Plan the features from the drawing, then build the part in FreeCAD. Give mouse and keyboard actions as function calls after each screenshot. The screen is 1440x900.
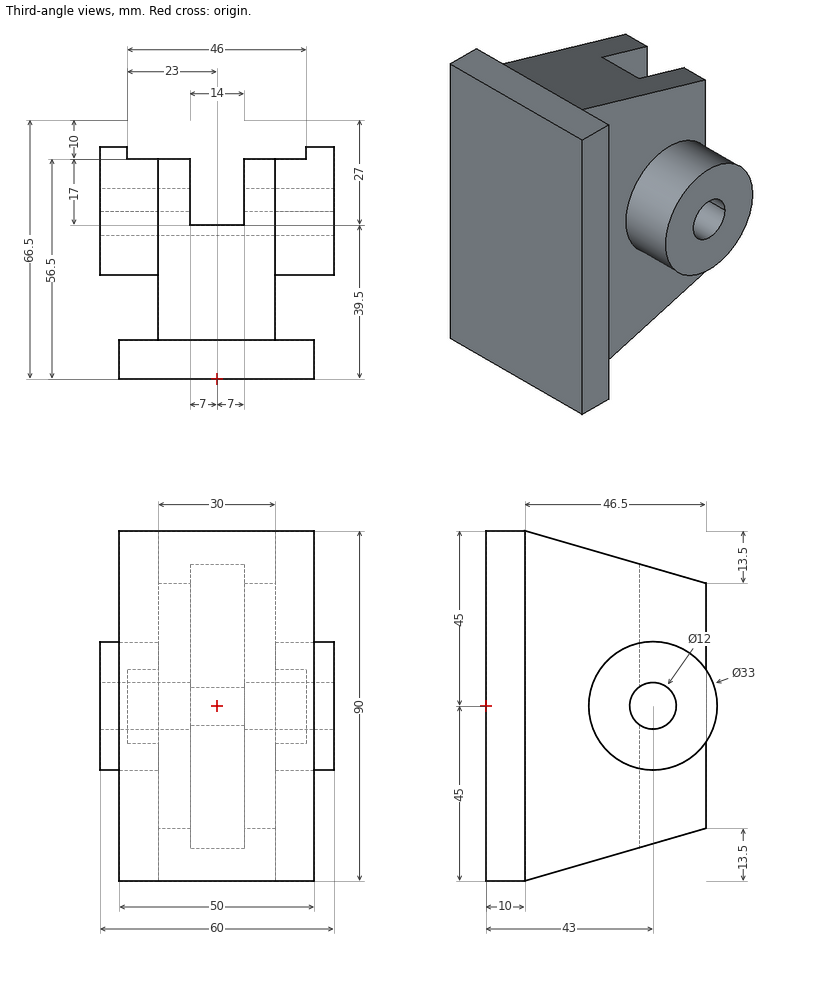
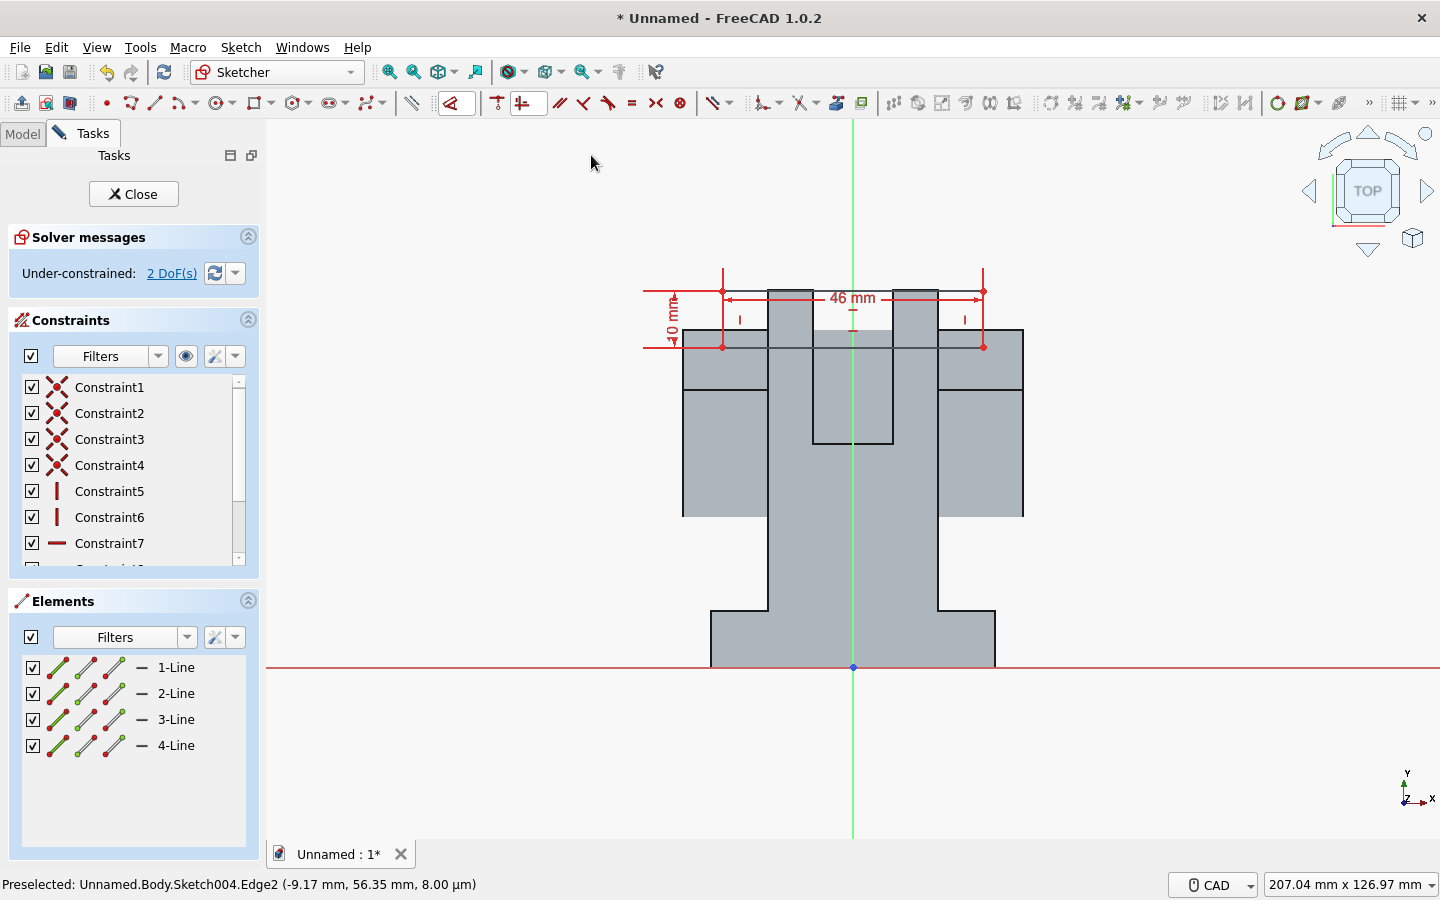
click(723, 291)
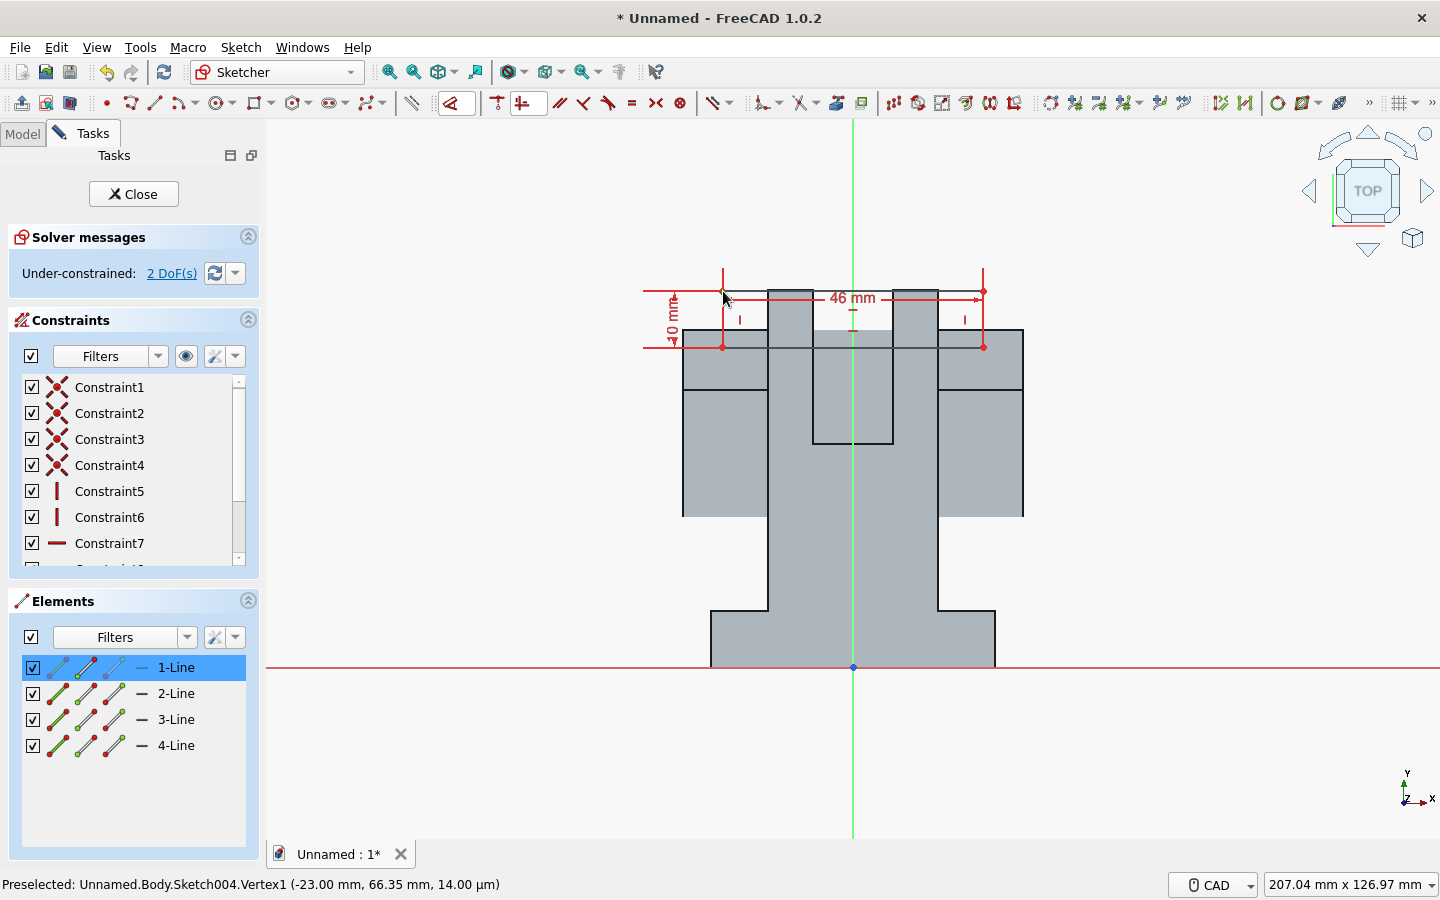
click(470, 104)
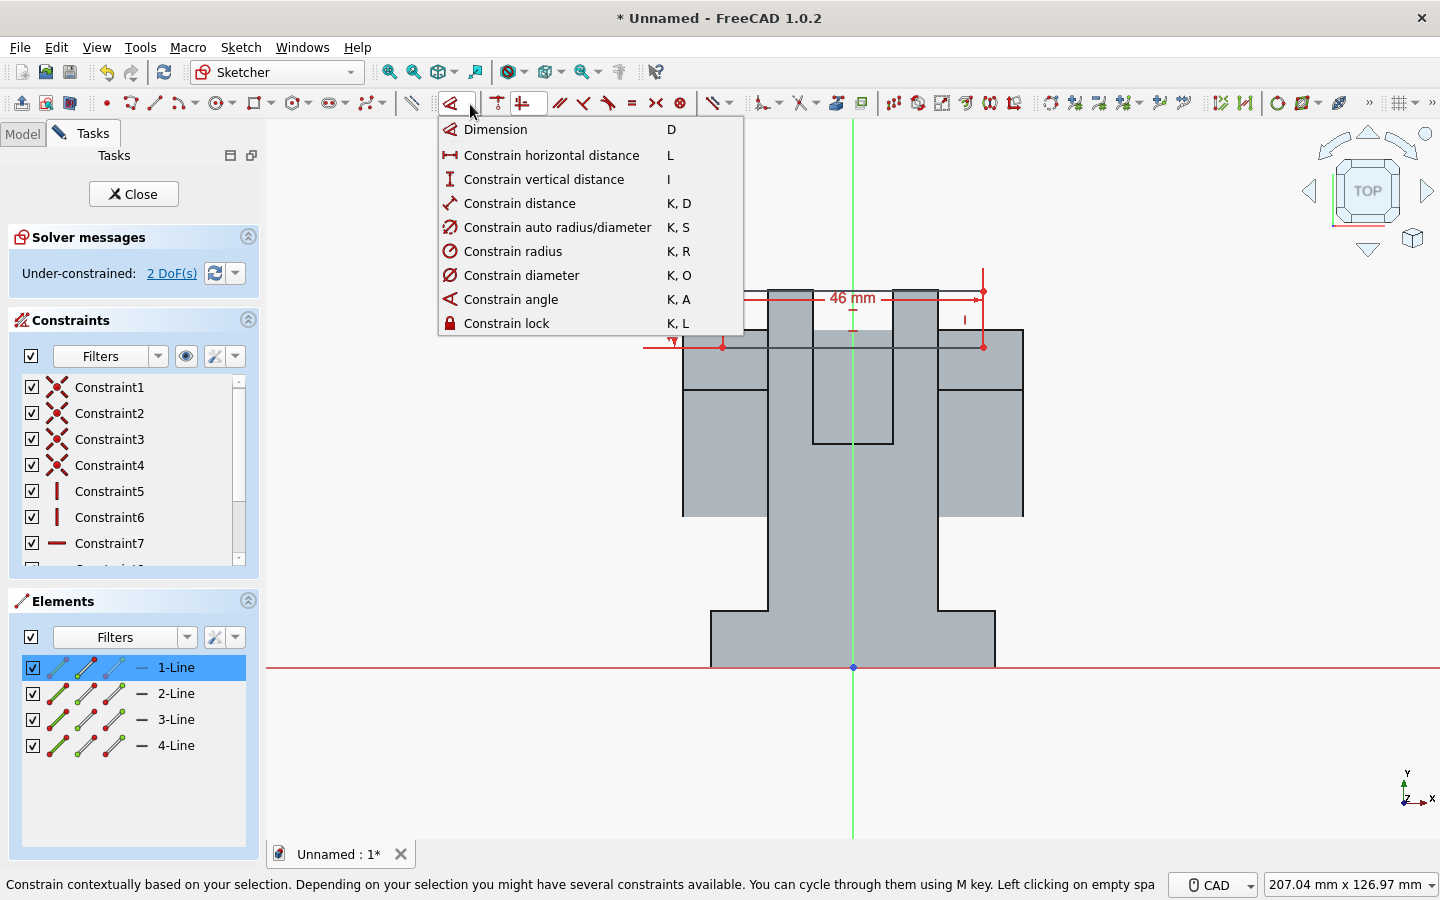
click(591, 155)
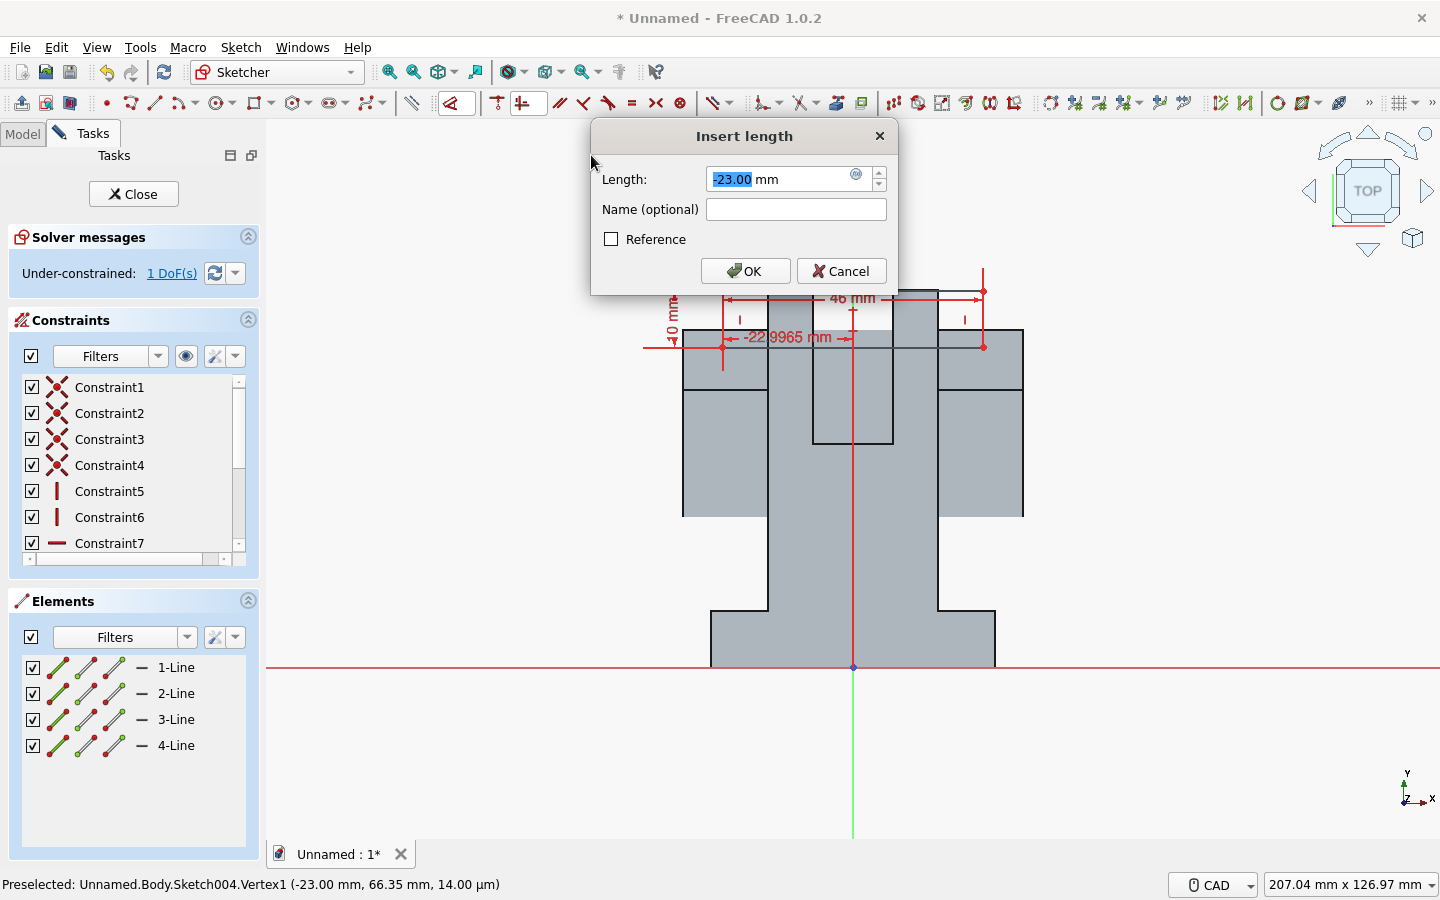
text(-23)
key(Return)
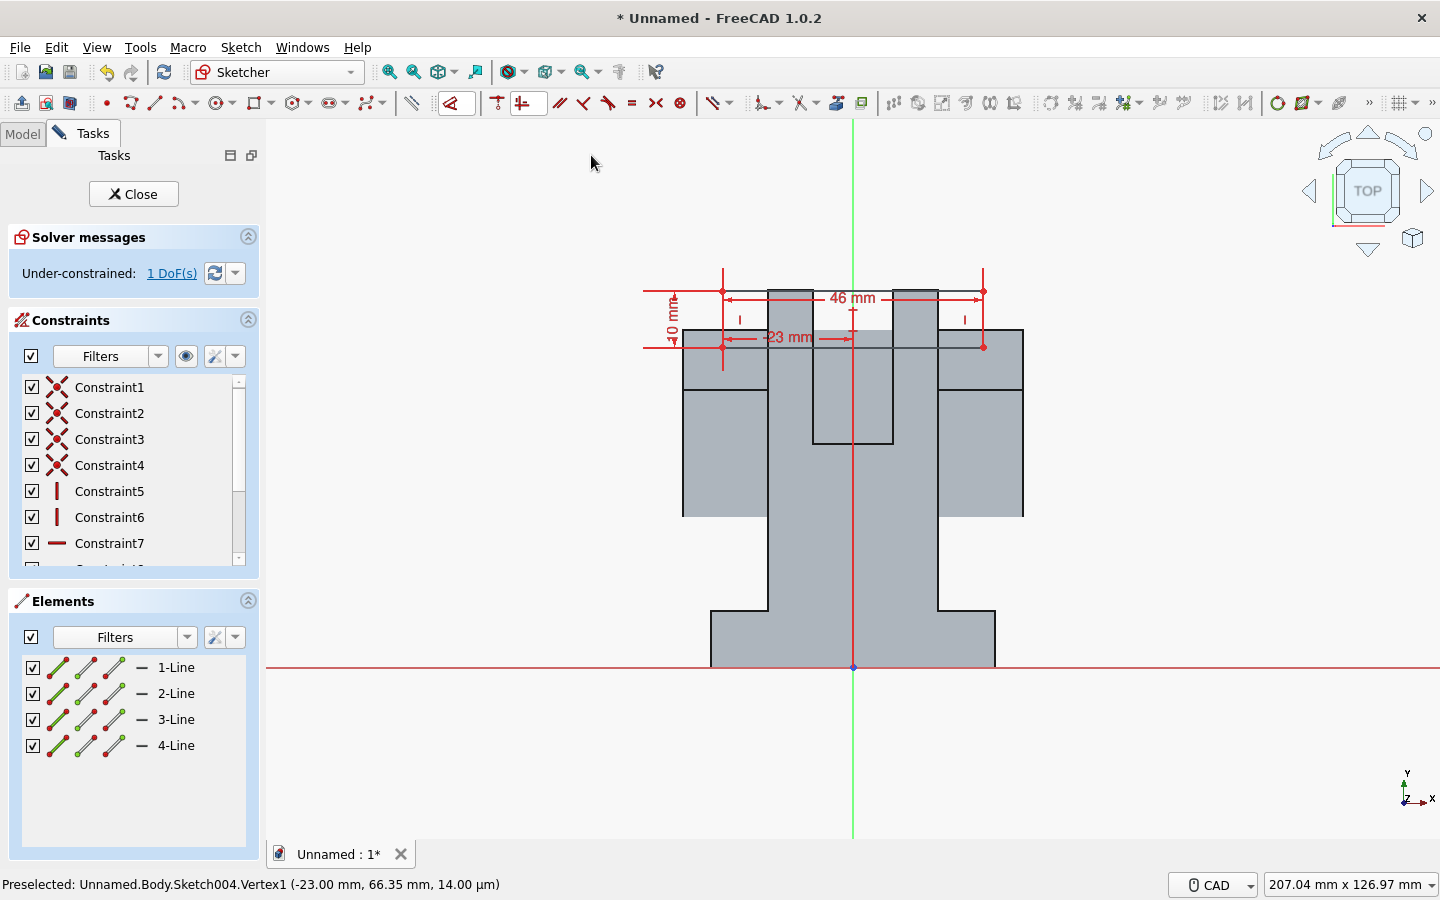
click(723, 291)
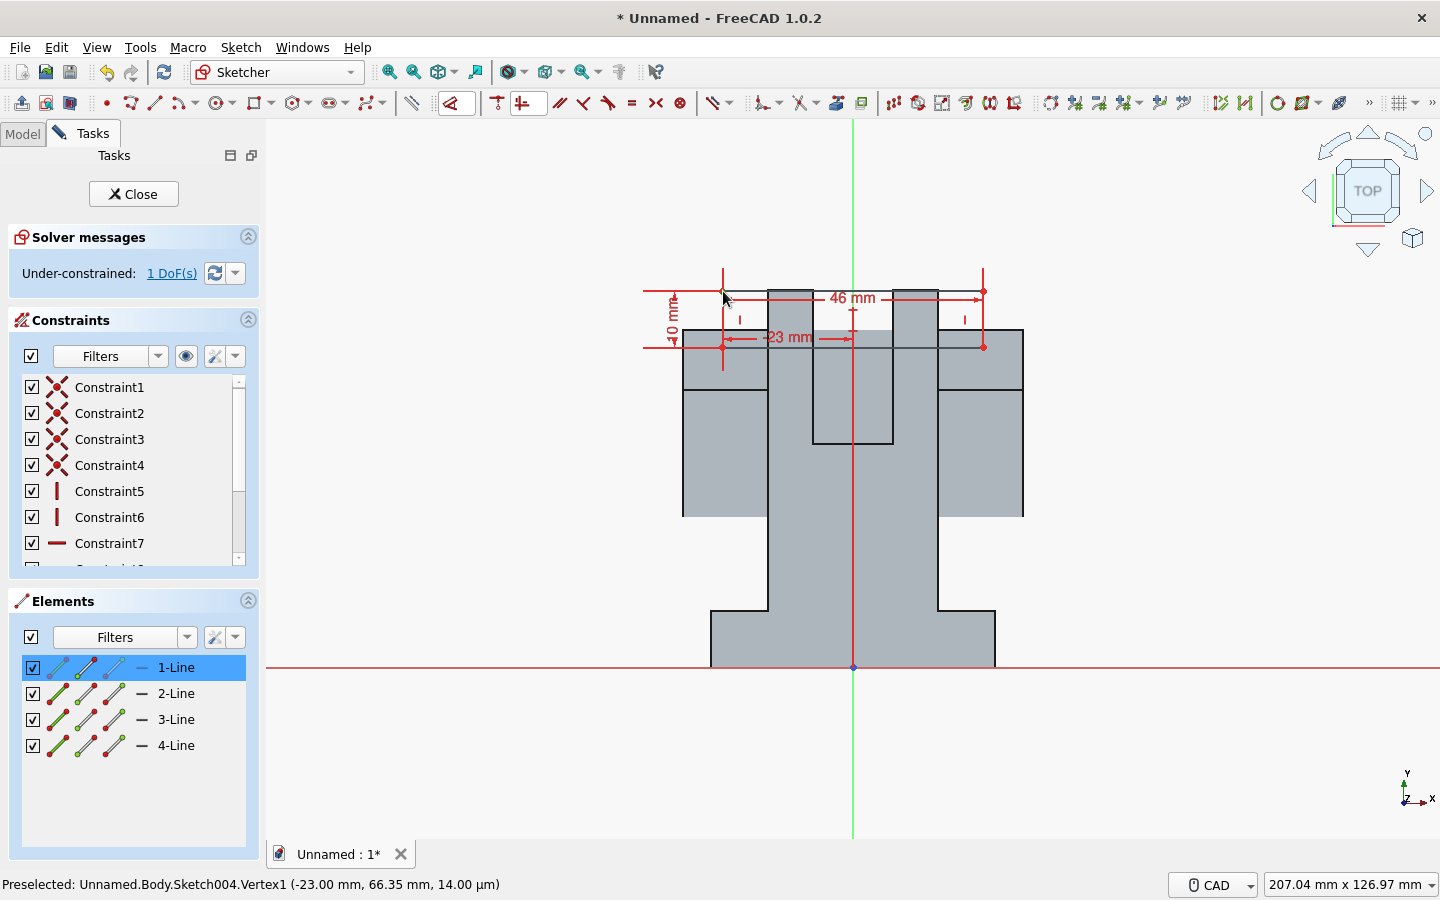
click(470, 104)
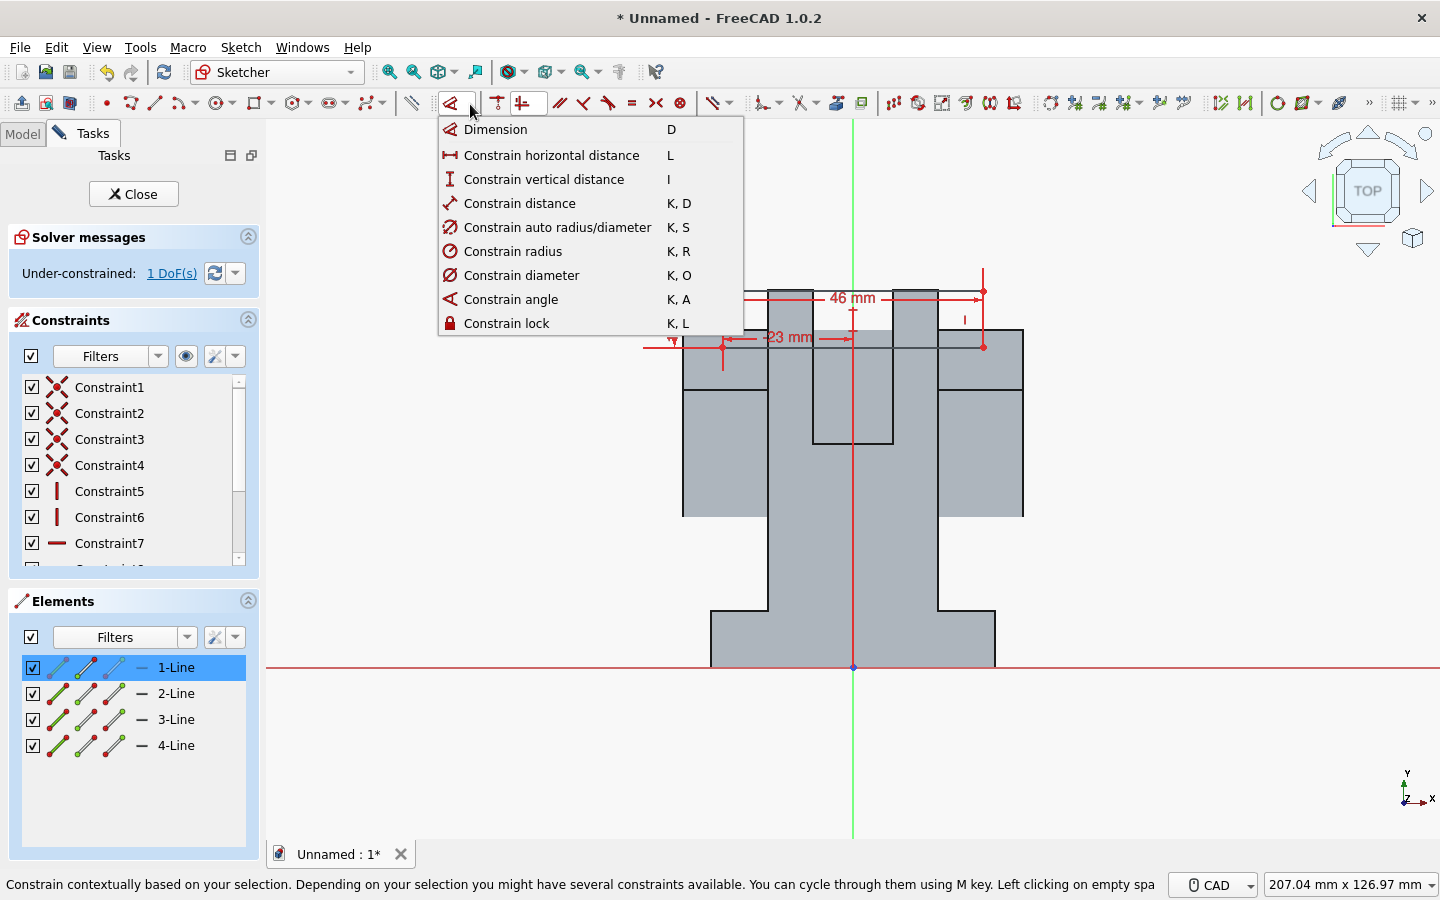
click(591, 179)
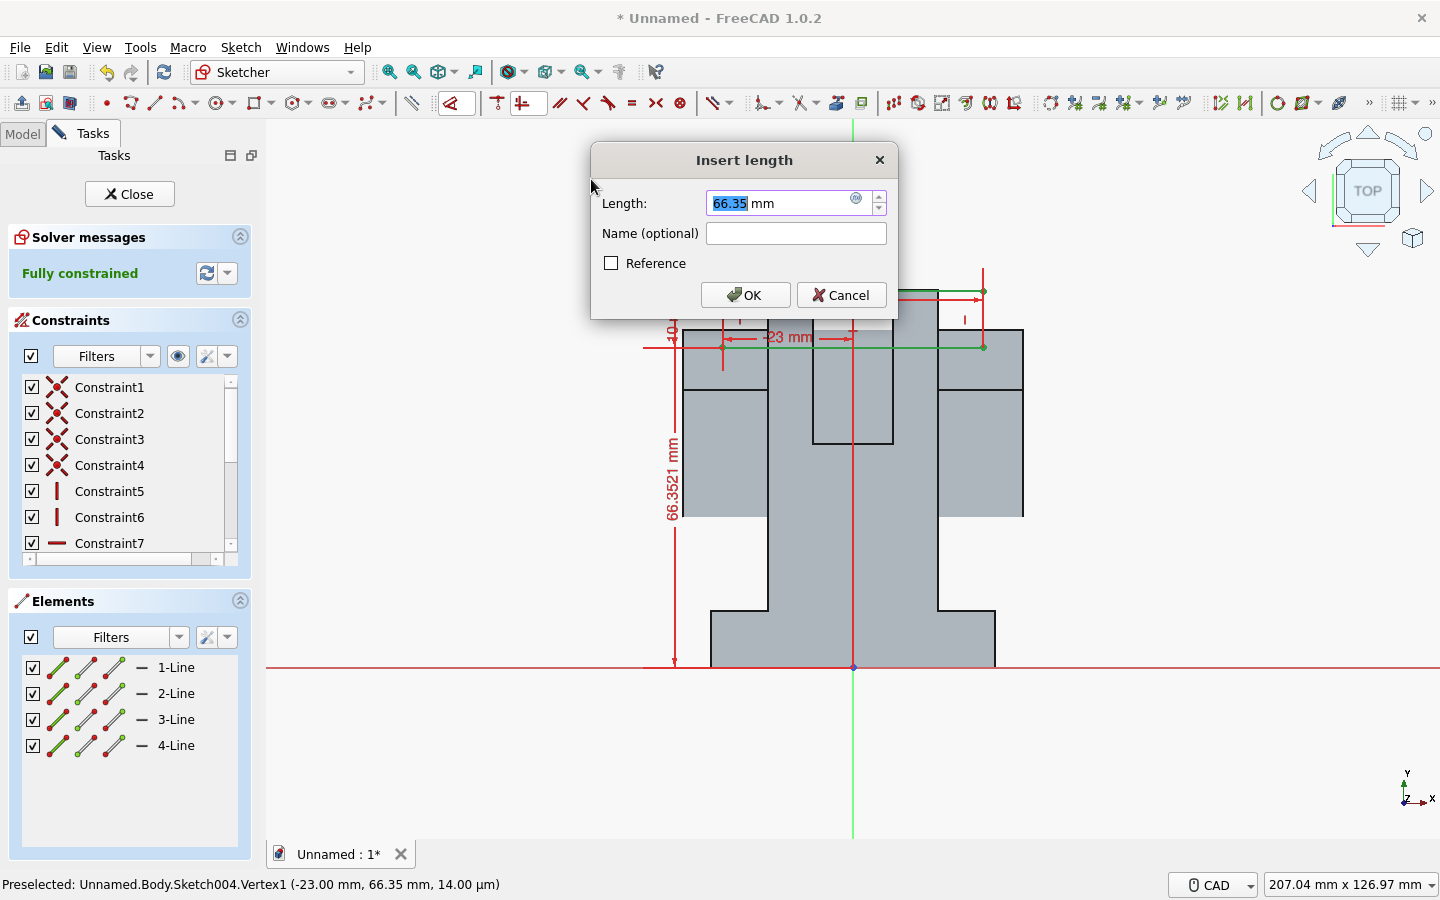
text(66.5)
key(Return)